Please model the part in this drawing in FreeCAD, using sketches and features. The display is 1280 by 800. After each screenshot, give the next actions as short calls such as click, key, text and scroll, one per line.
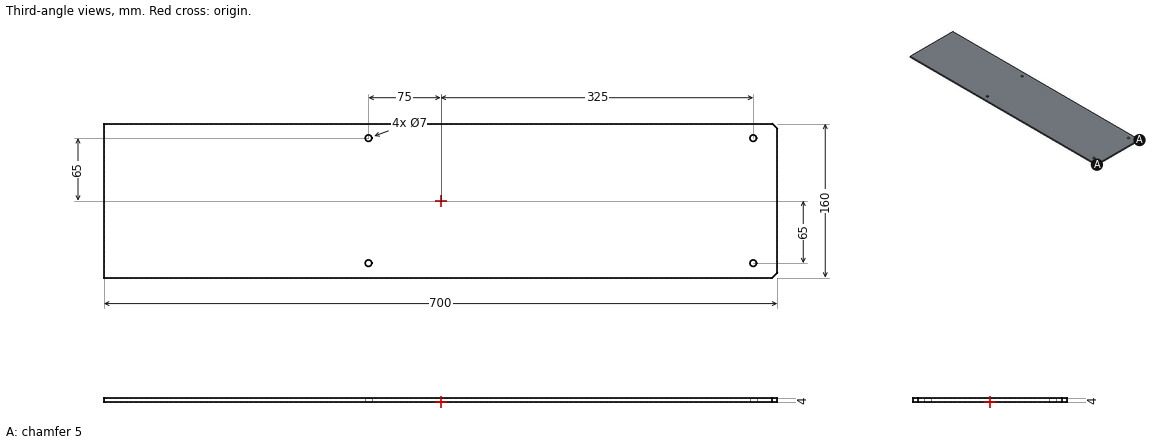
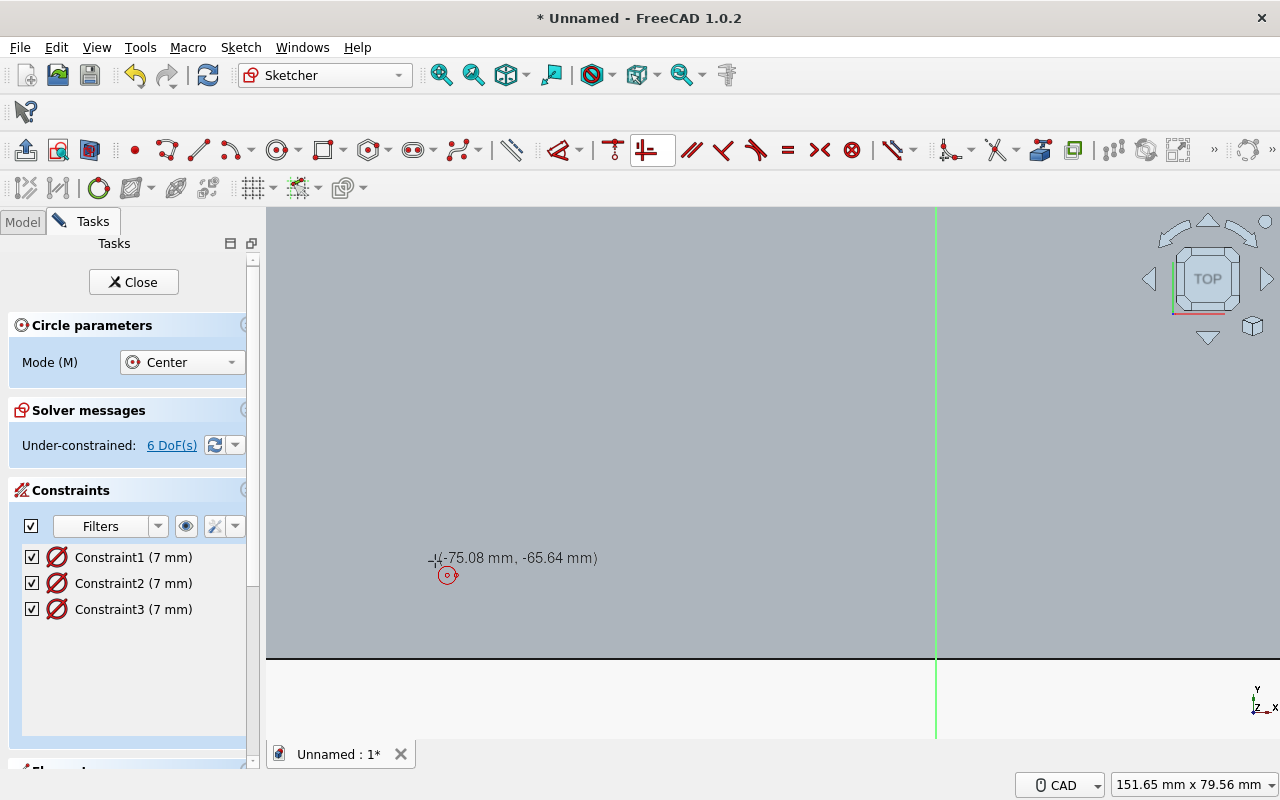
scroll(434, 561, down, 8)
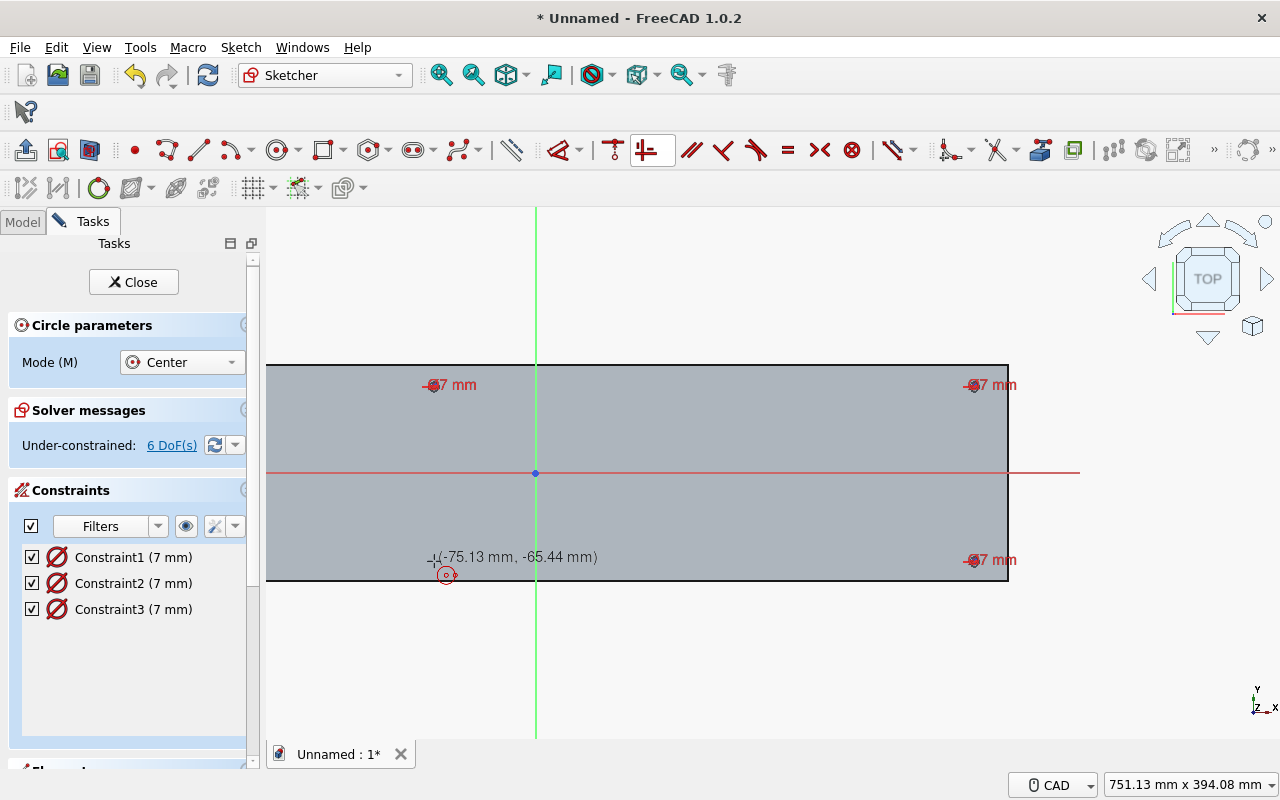
click(434, 561)
move(438, 558)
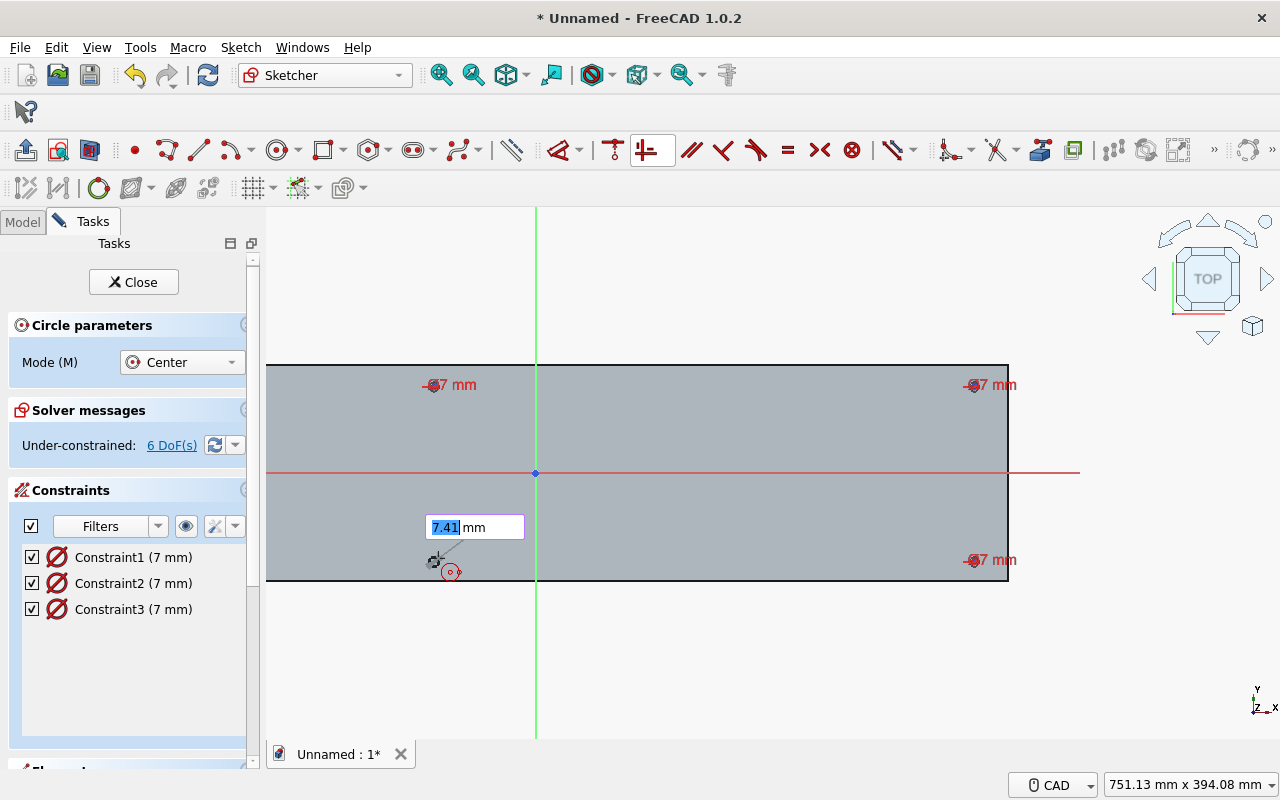
text(7)
key(Return)
key(Escape)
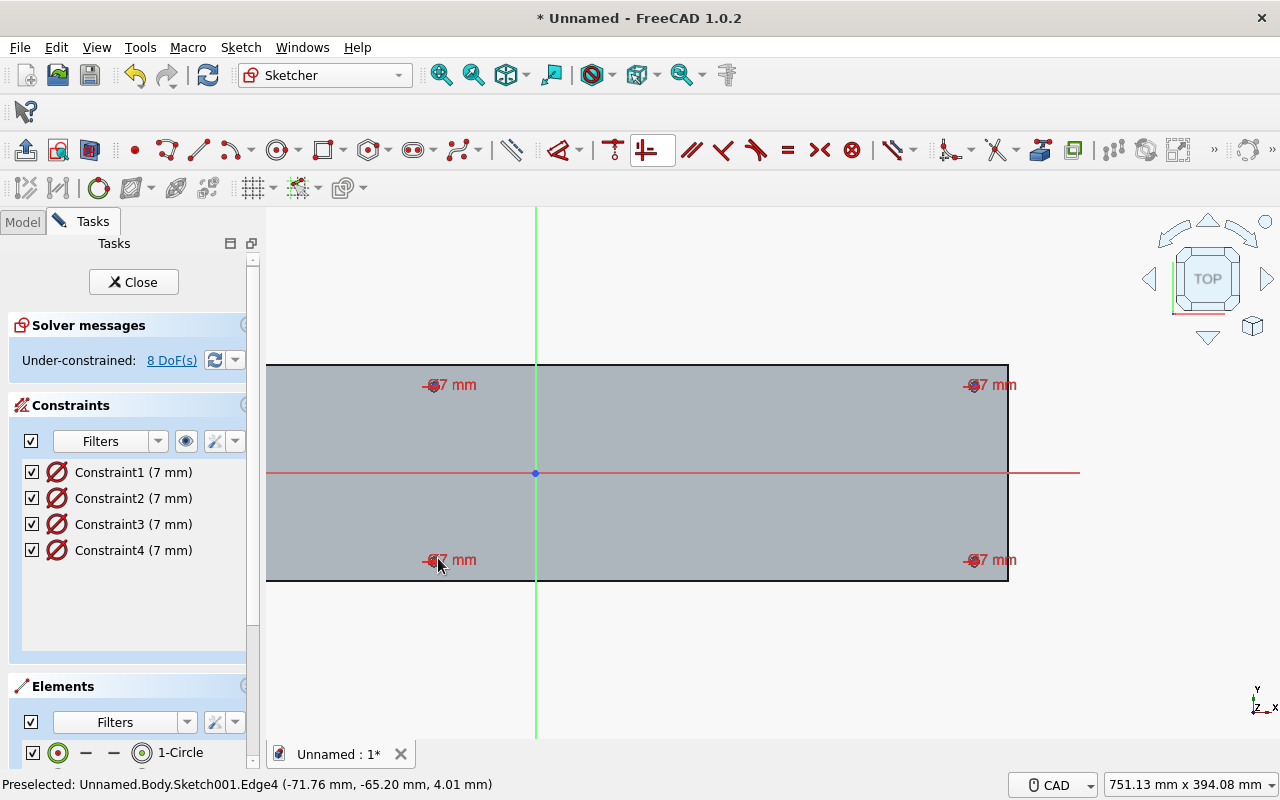
click(434, 387)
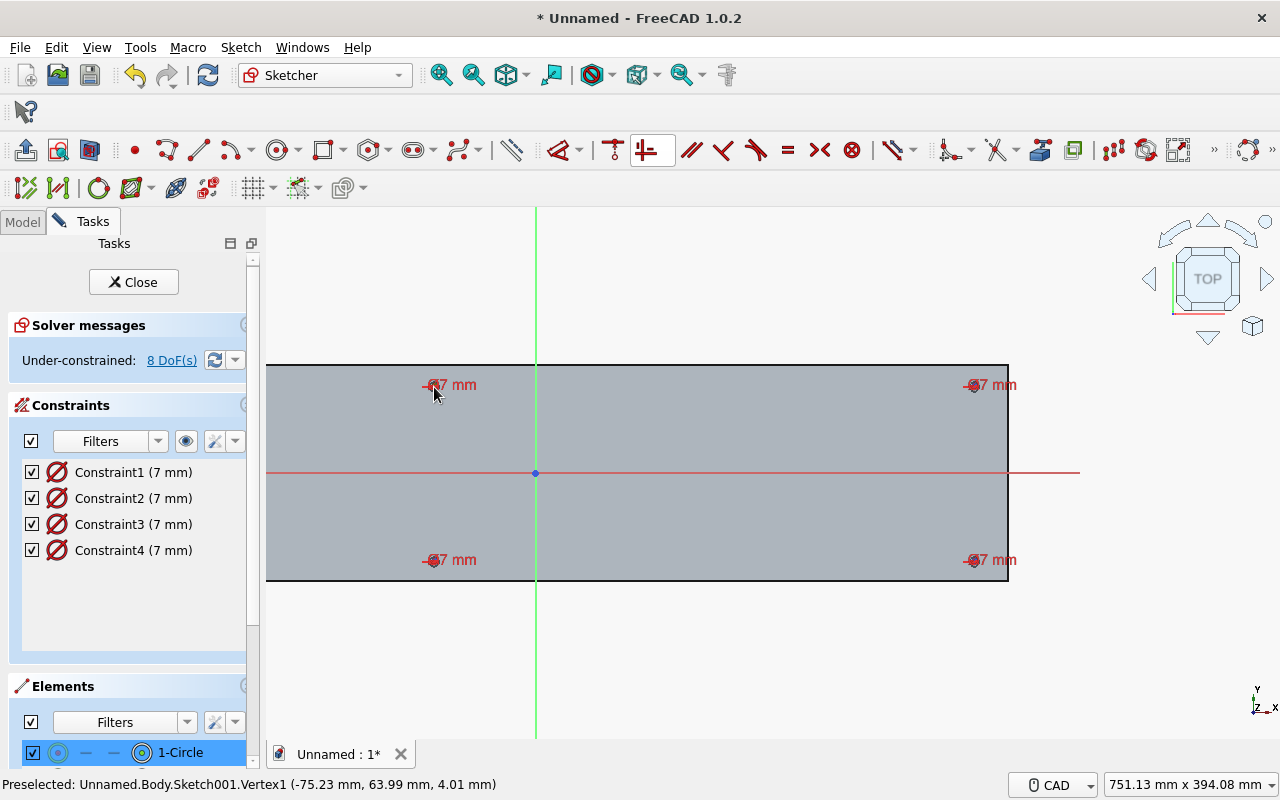
click(582, 150)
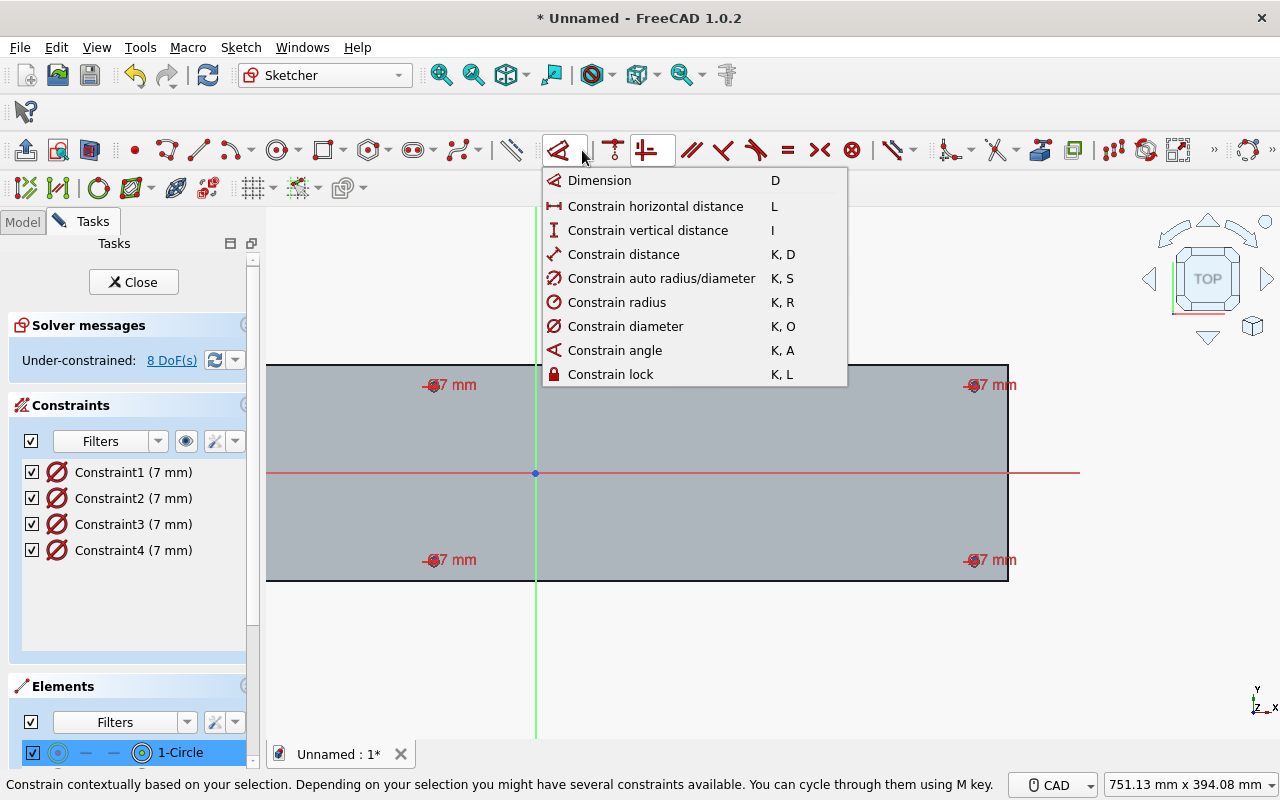
click(695, 206)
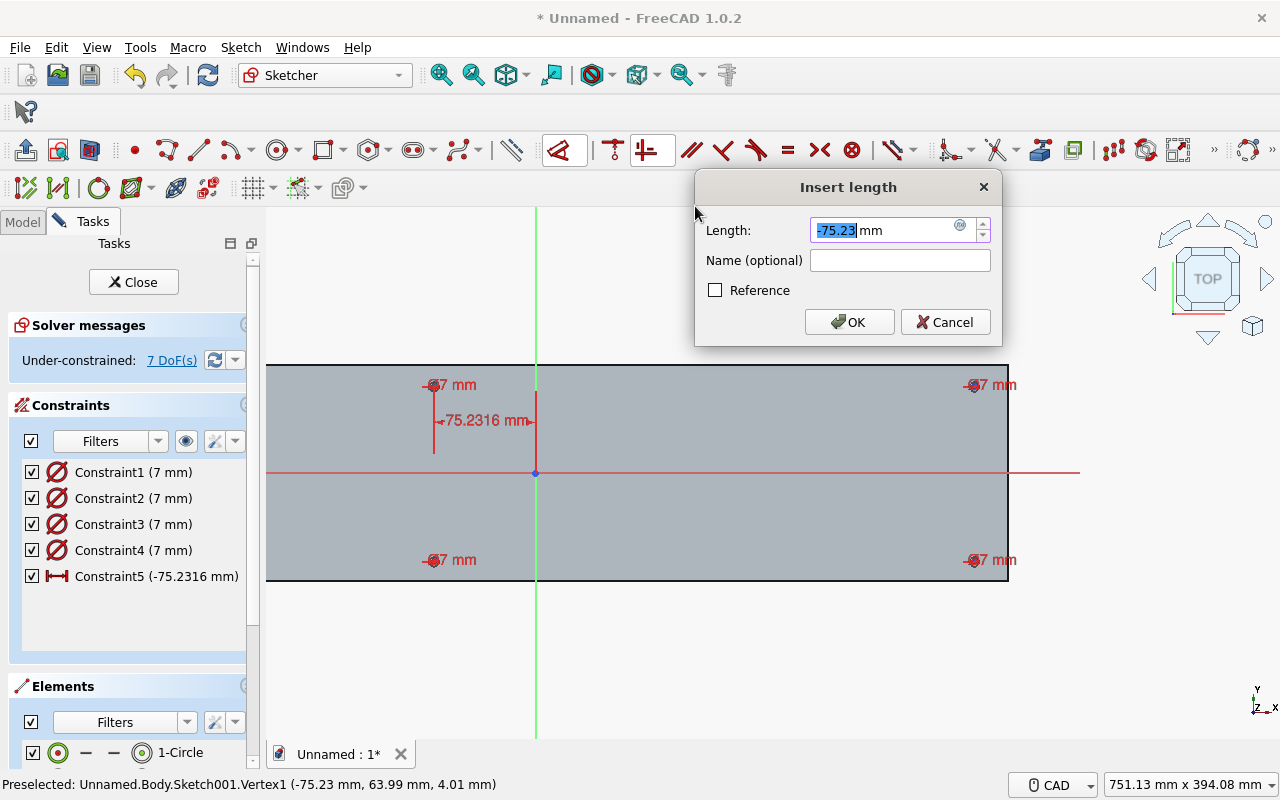
text(-75)
key(Return)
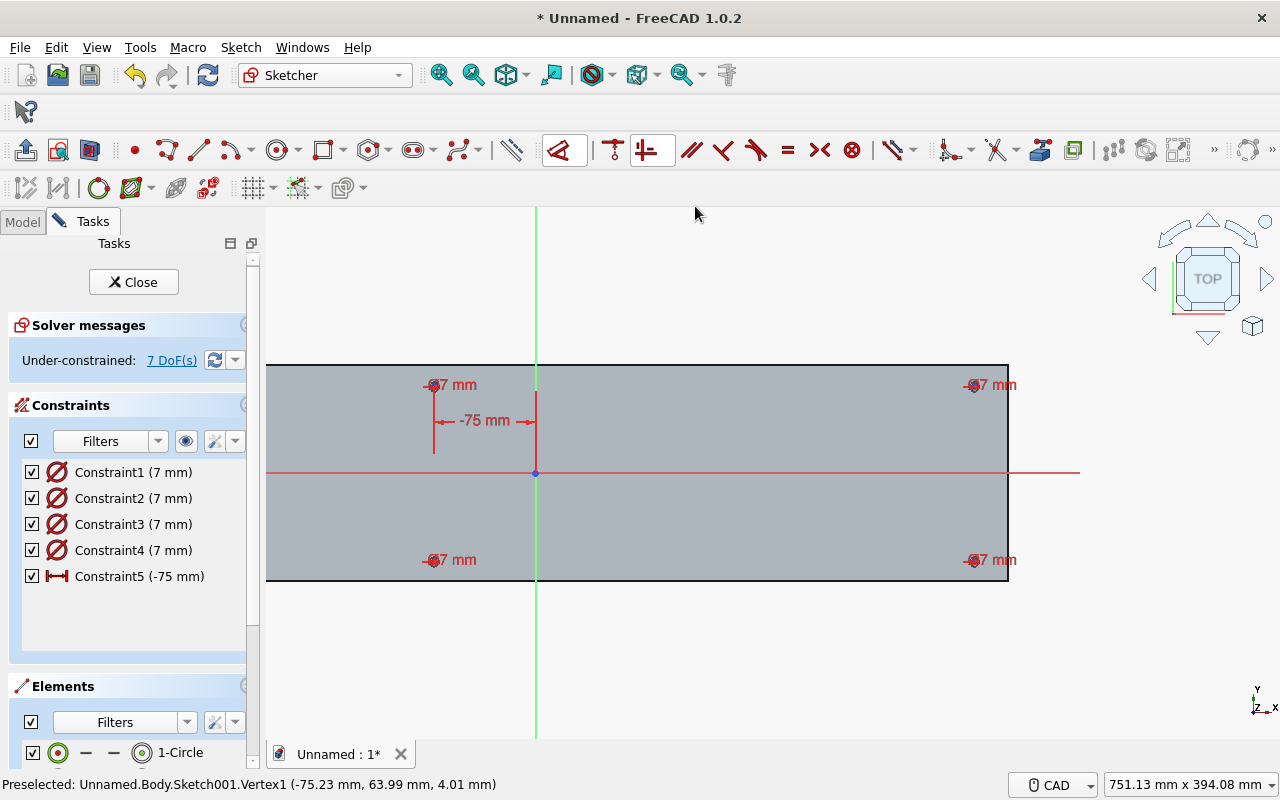
click(434, 387)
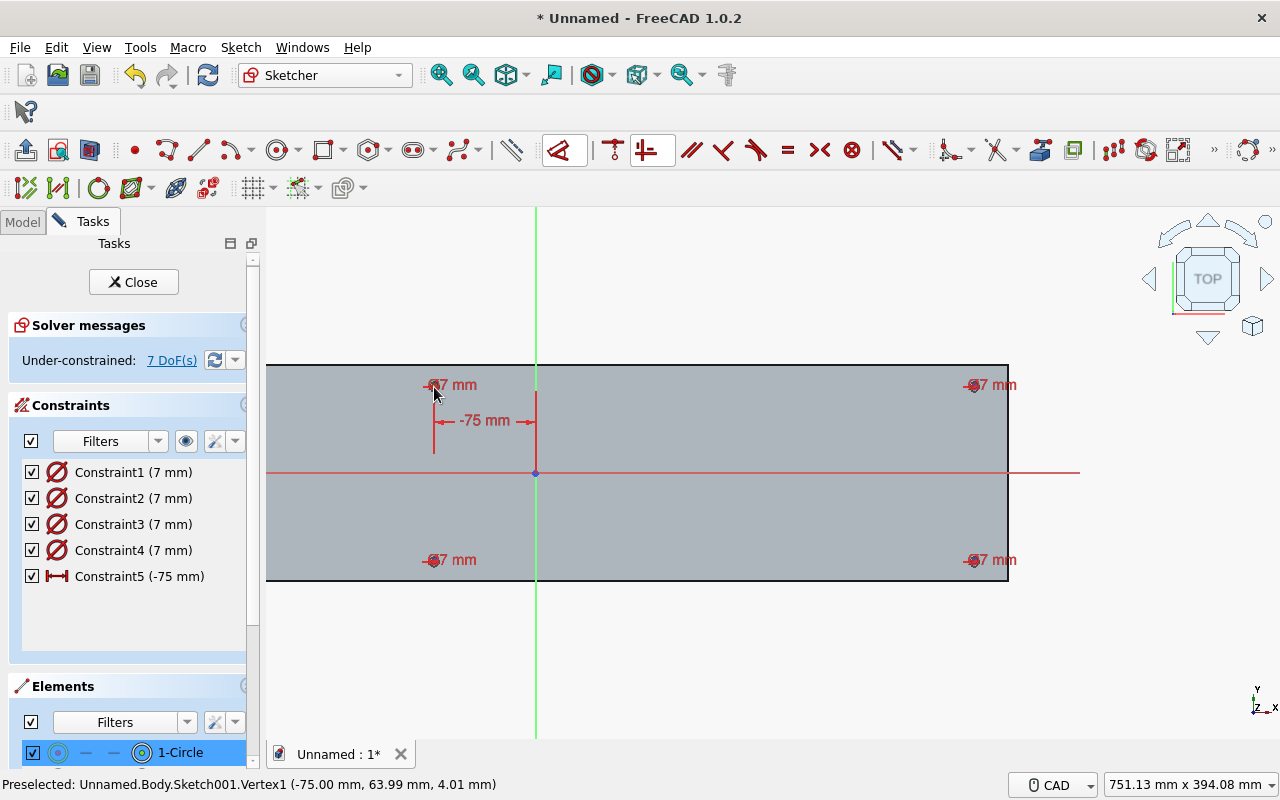
key(i)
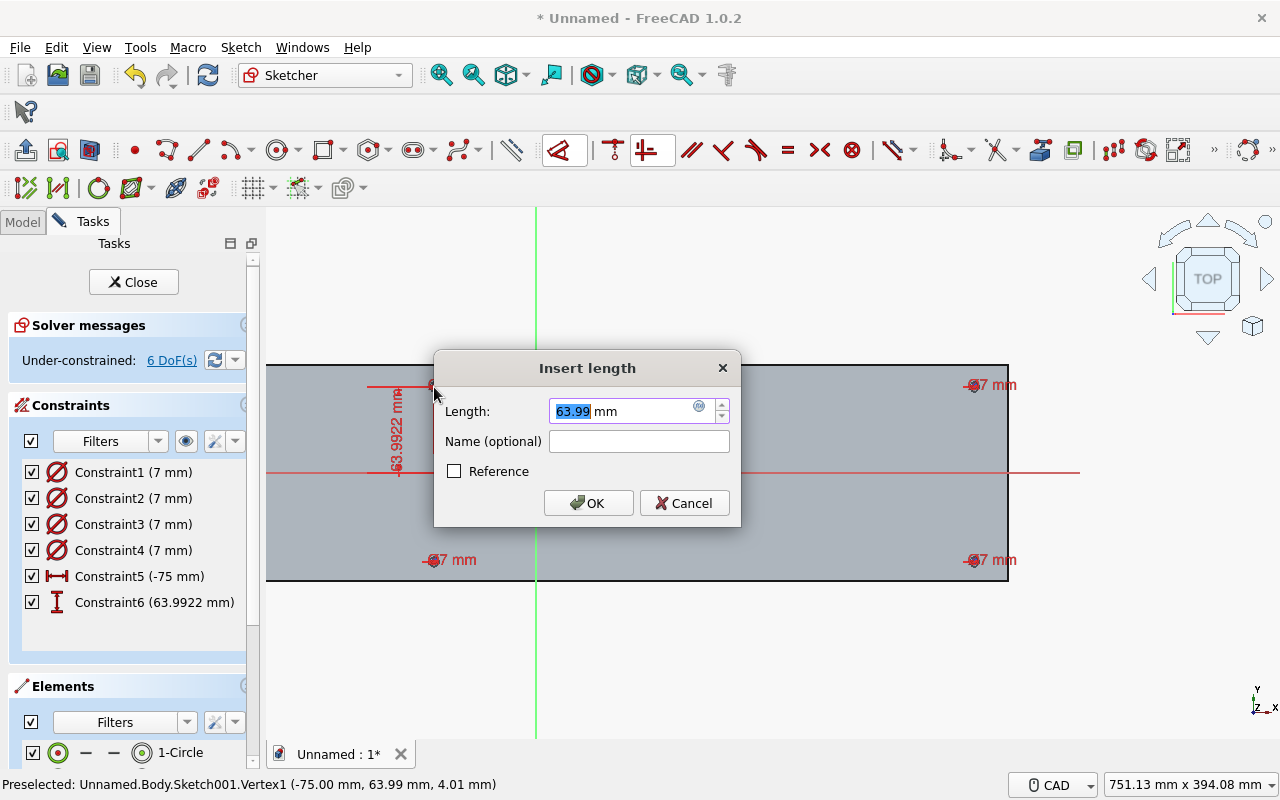
text(65)
key(Return)